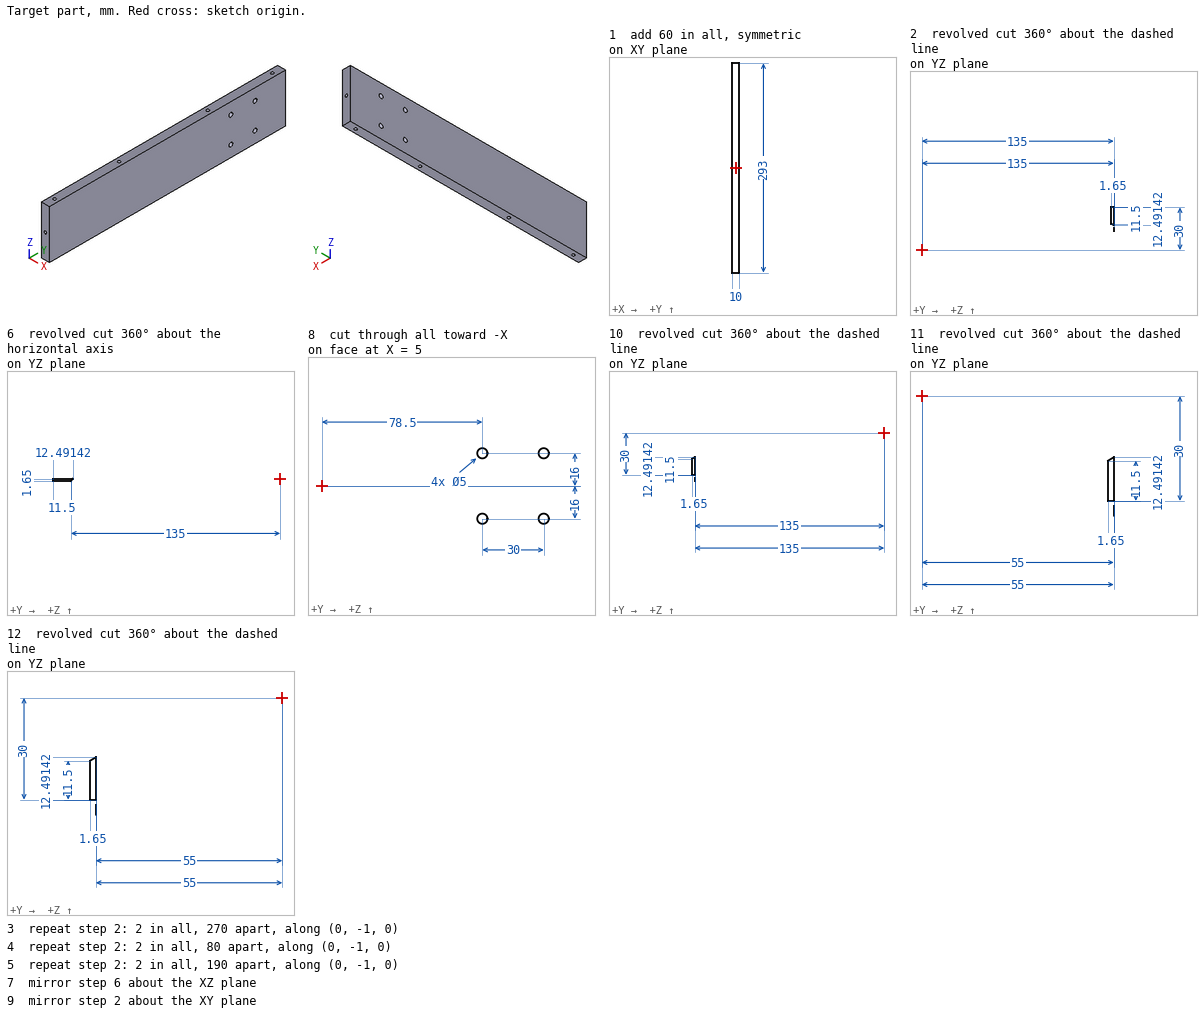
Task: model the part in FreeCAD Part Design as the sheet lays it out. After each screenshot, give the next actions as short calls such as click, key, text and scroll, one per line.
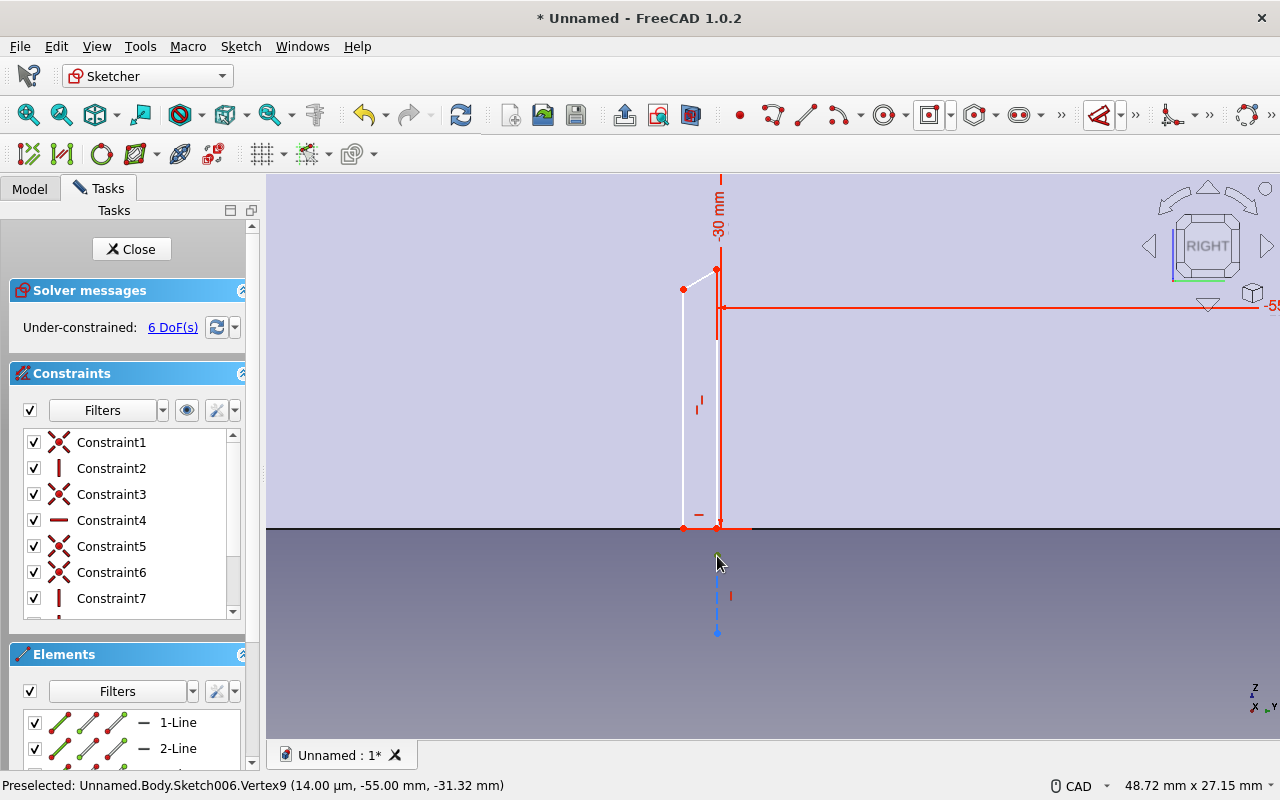
click(1120, 116)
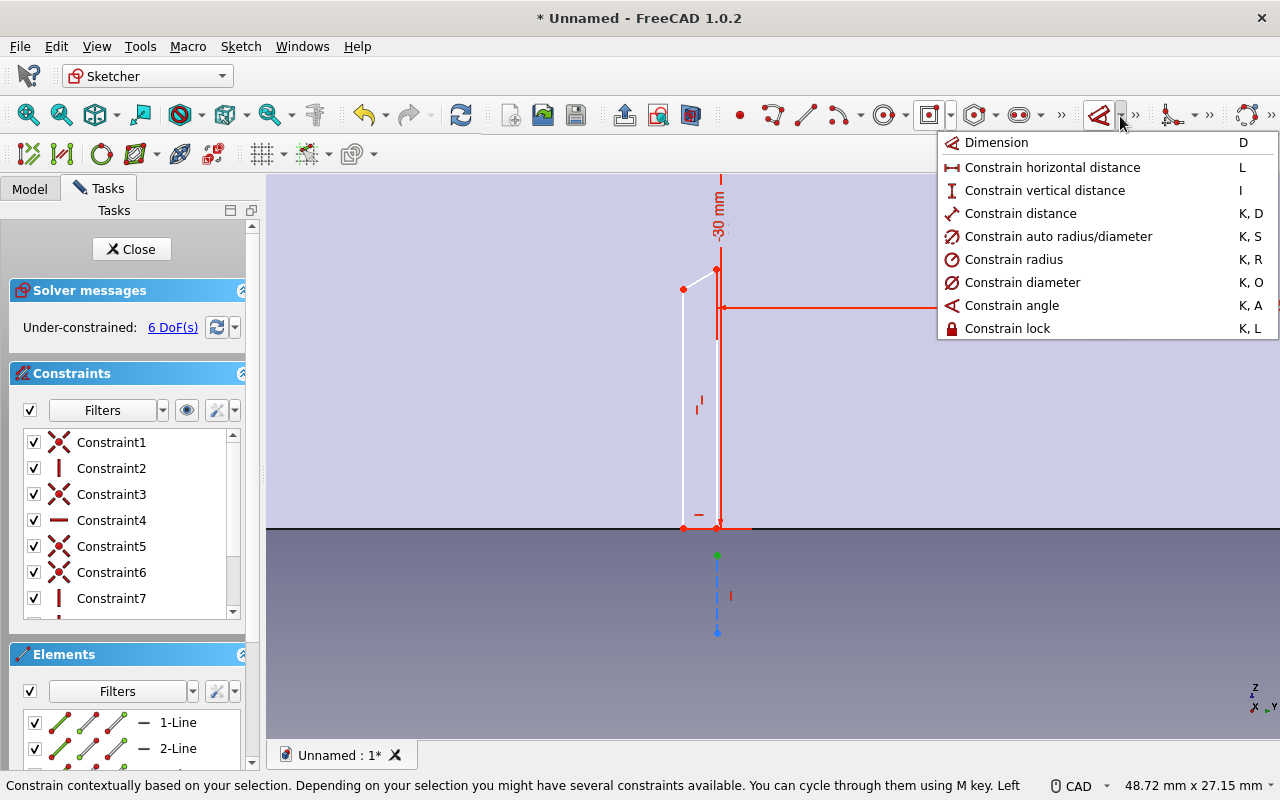
click(1108, 168)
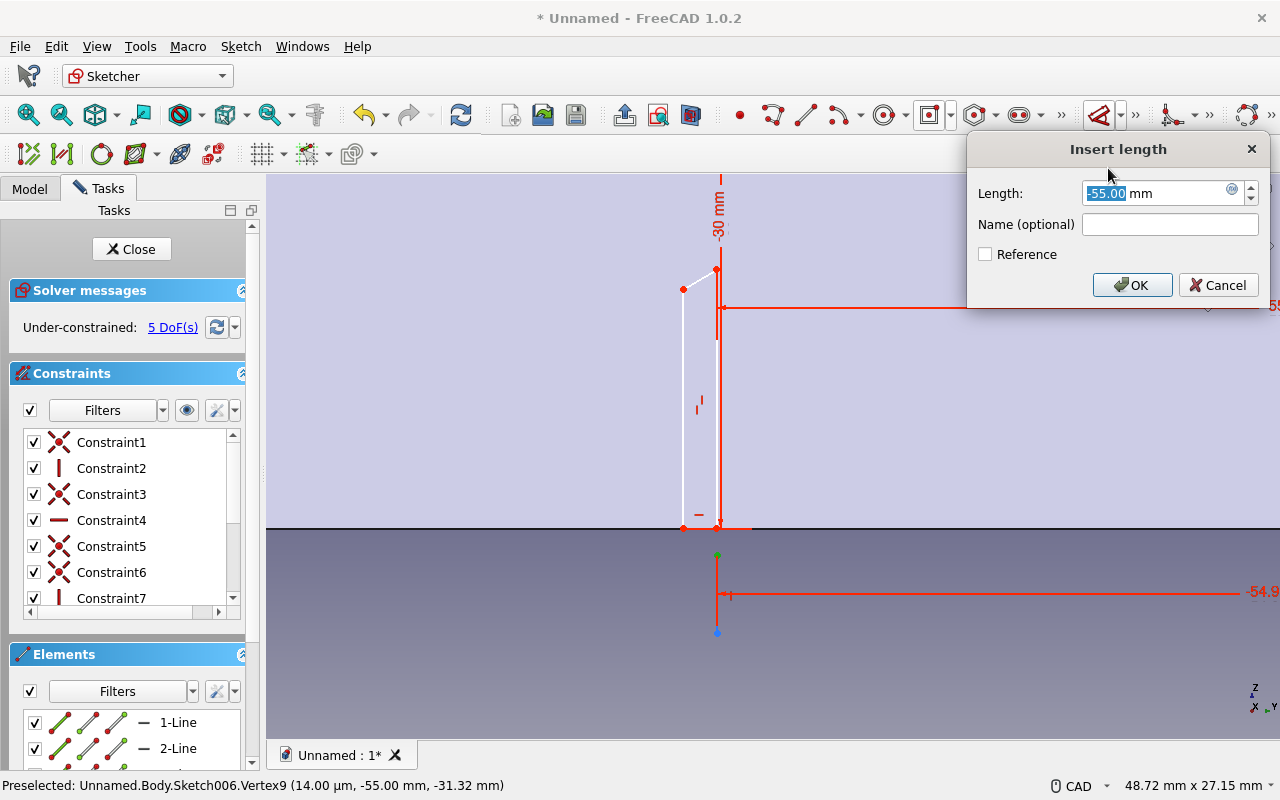
text(-55)
key(Return)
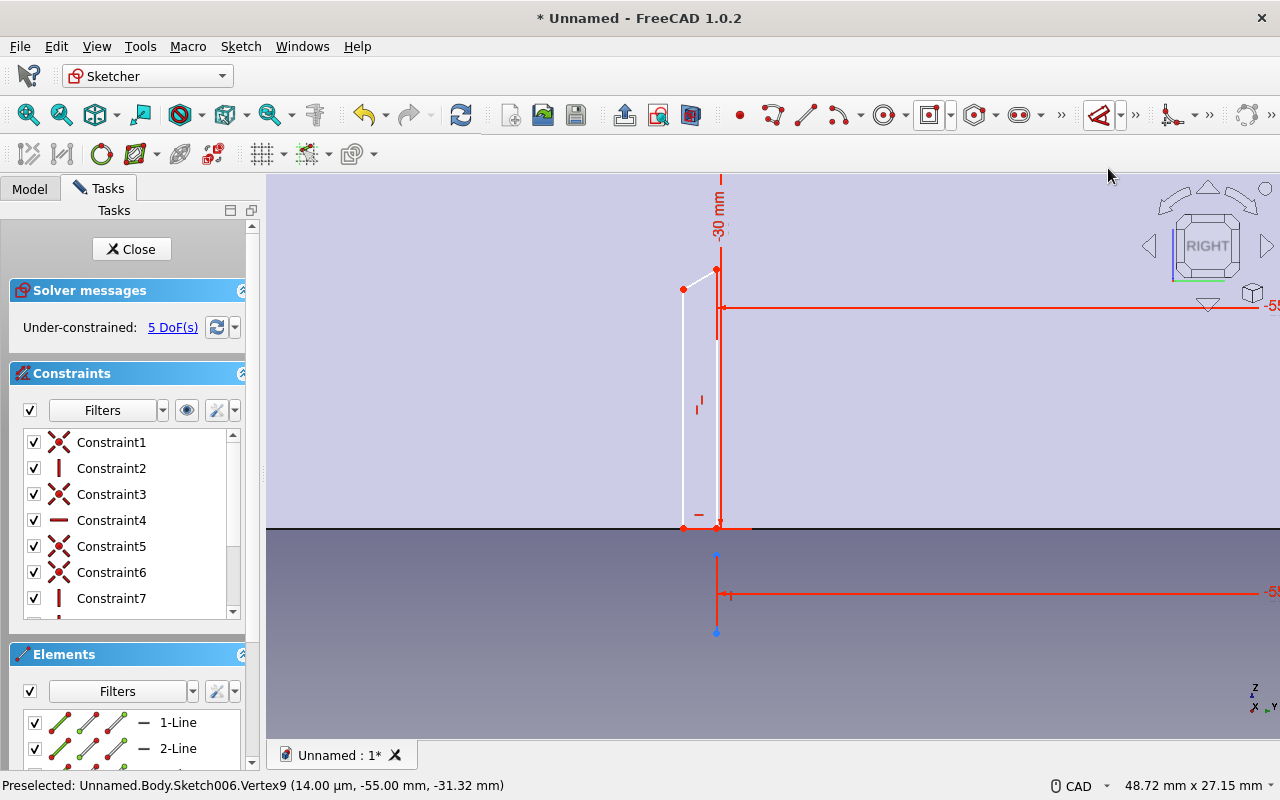
click(683, 362)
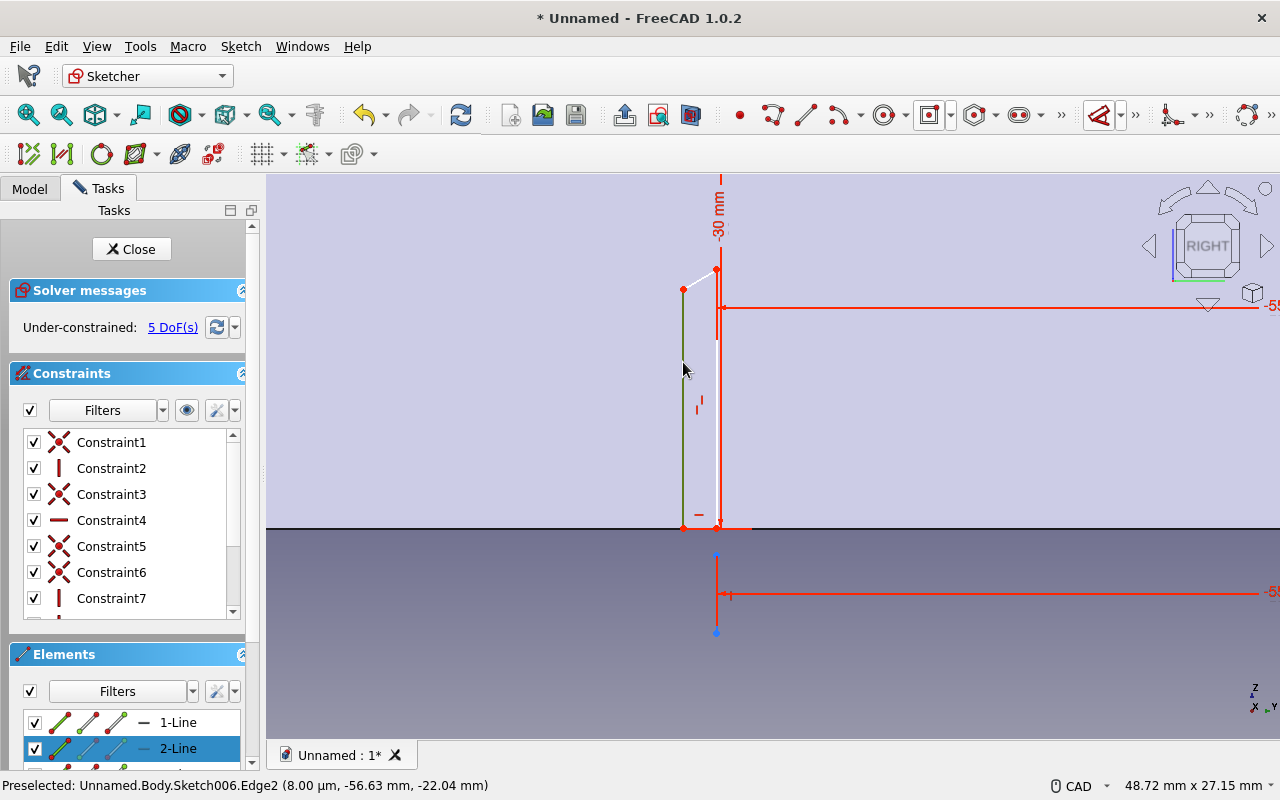
click(1120, 116)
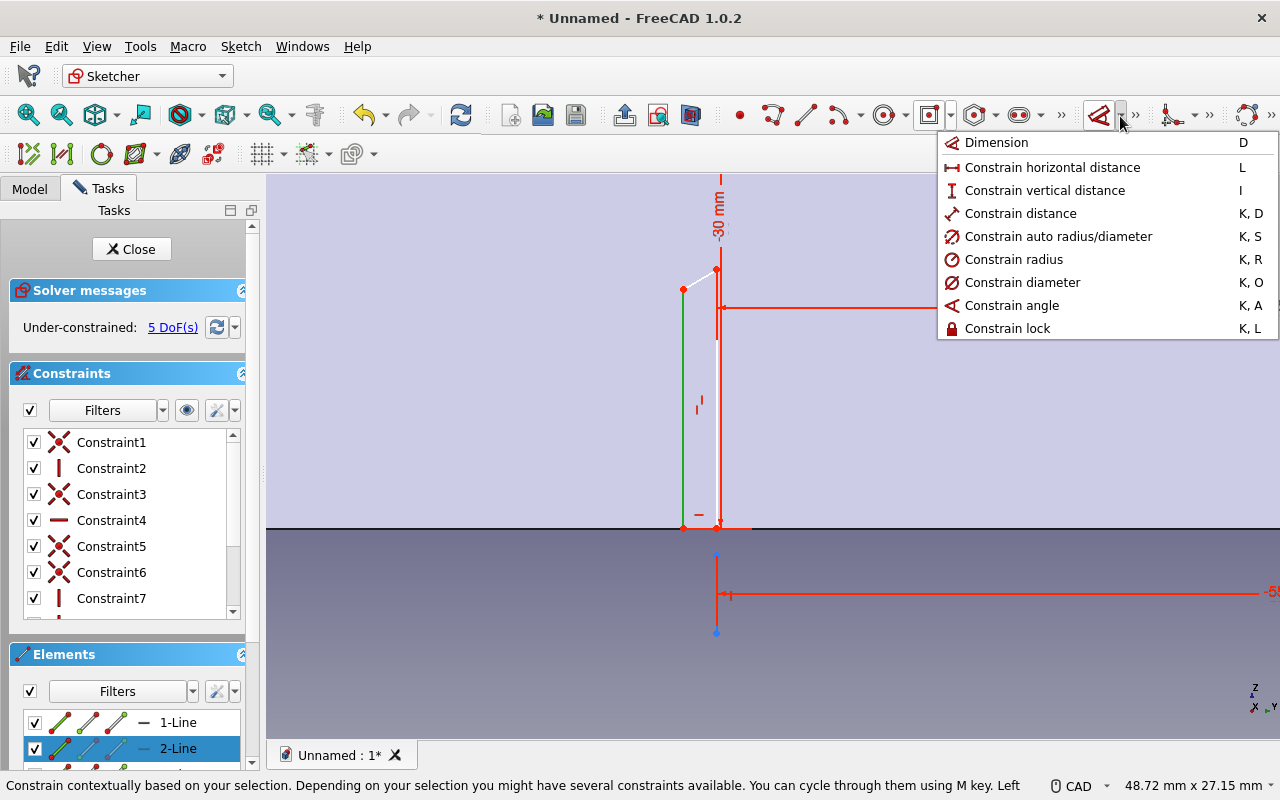
click(1108, 190)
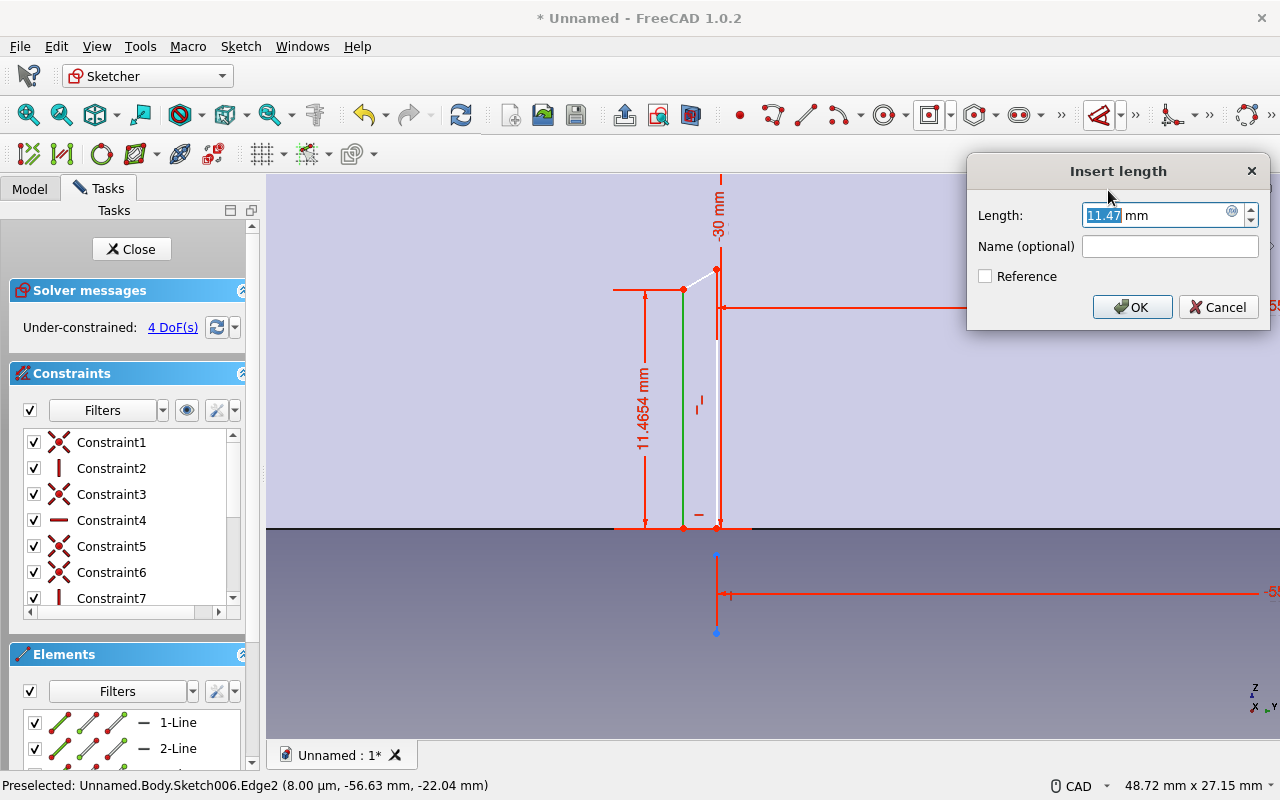
text(11.5)
key(Return)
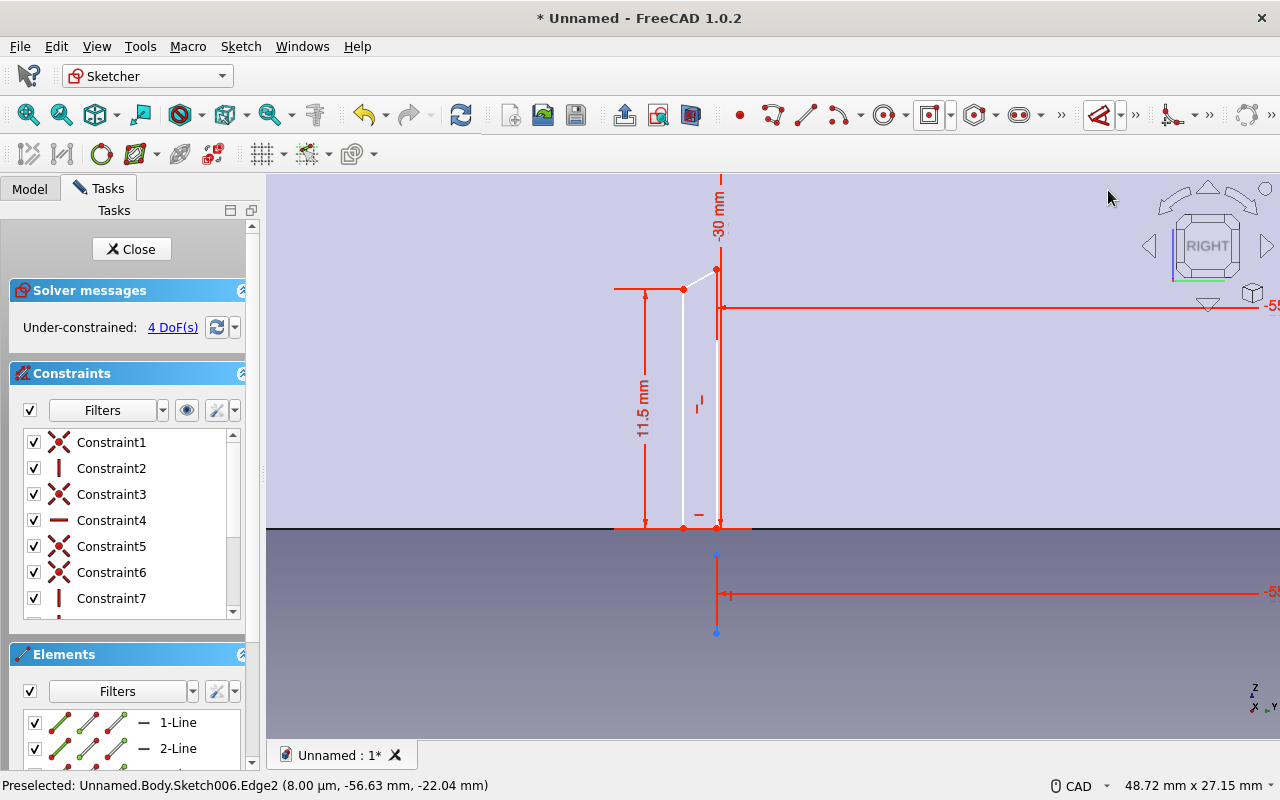
scroll(693, 529, up, 2)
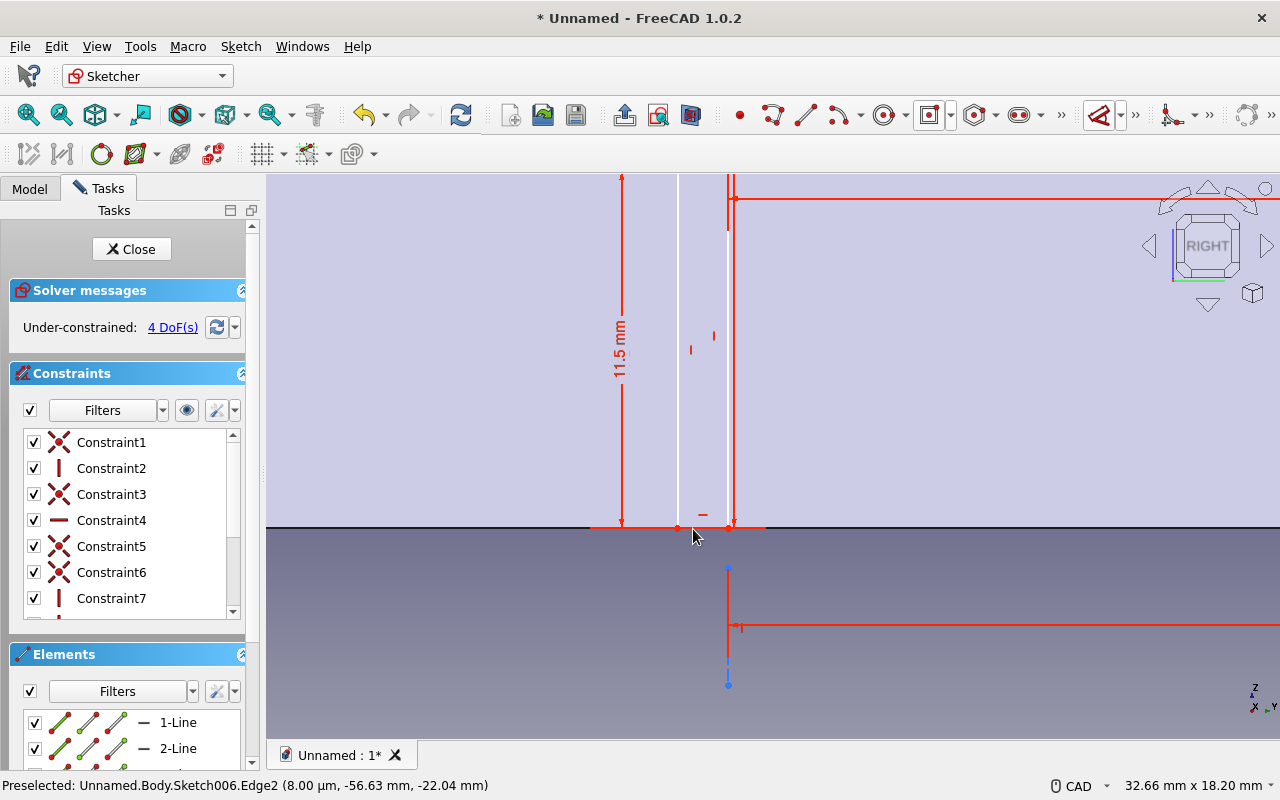
click(693, 528)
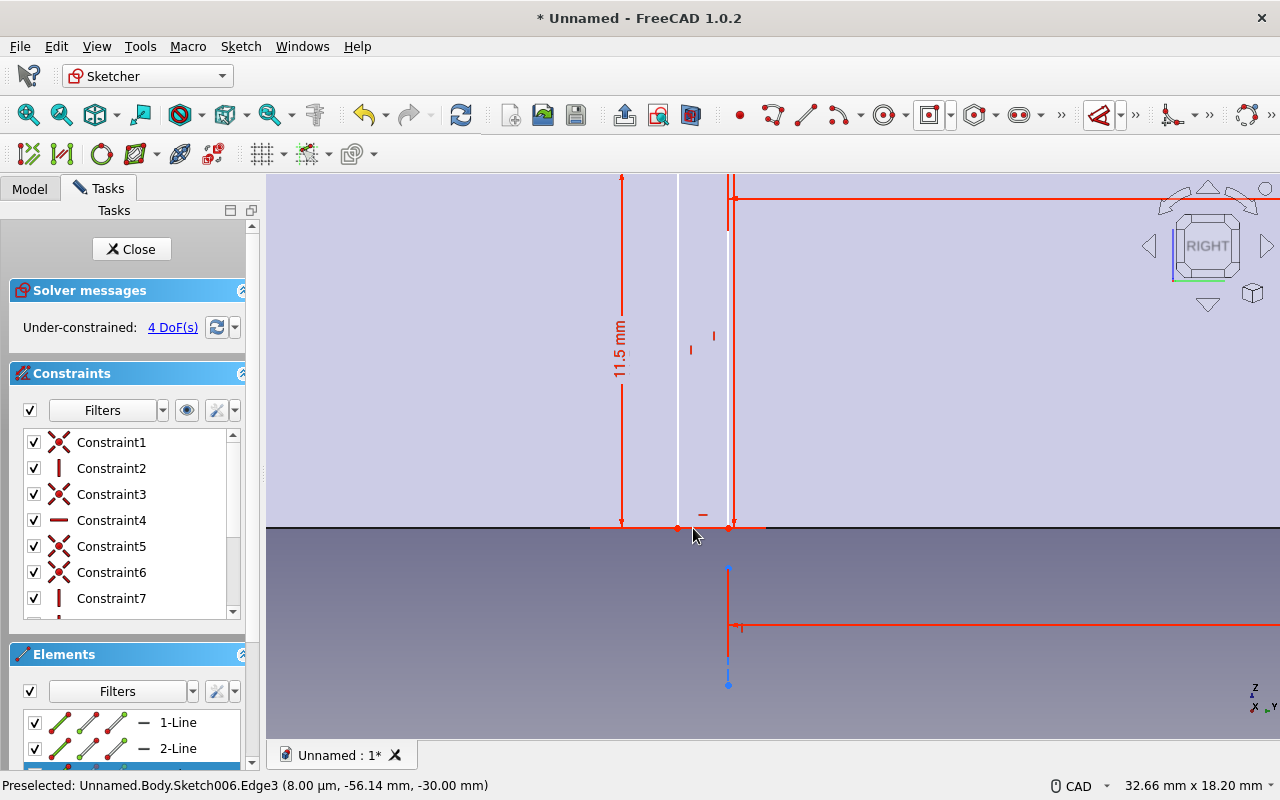
key(l)